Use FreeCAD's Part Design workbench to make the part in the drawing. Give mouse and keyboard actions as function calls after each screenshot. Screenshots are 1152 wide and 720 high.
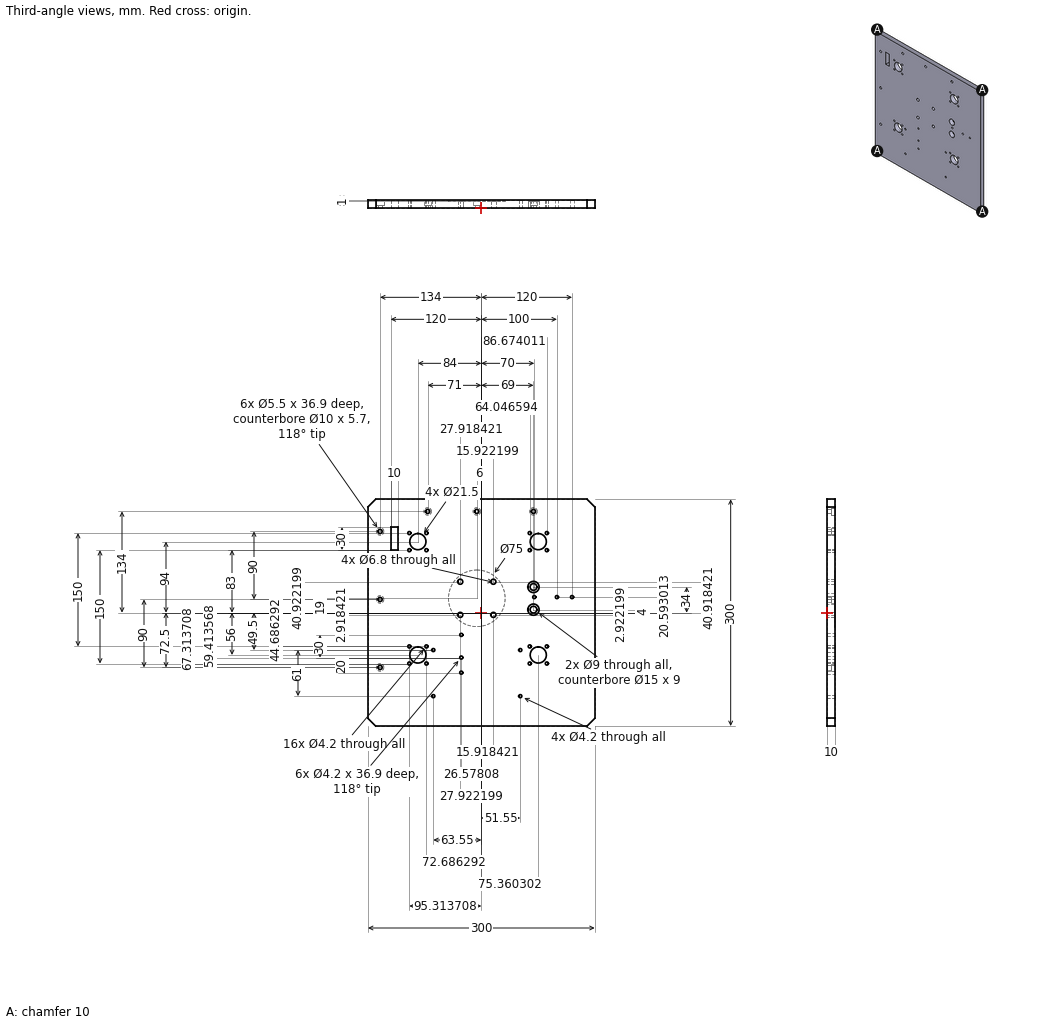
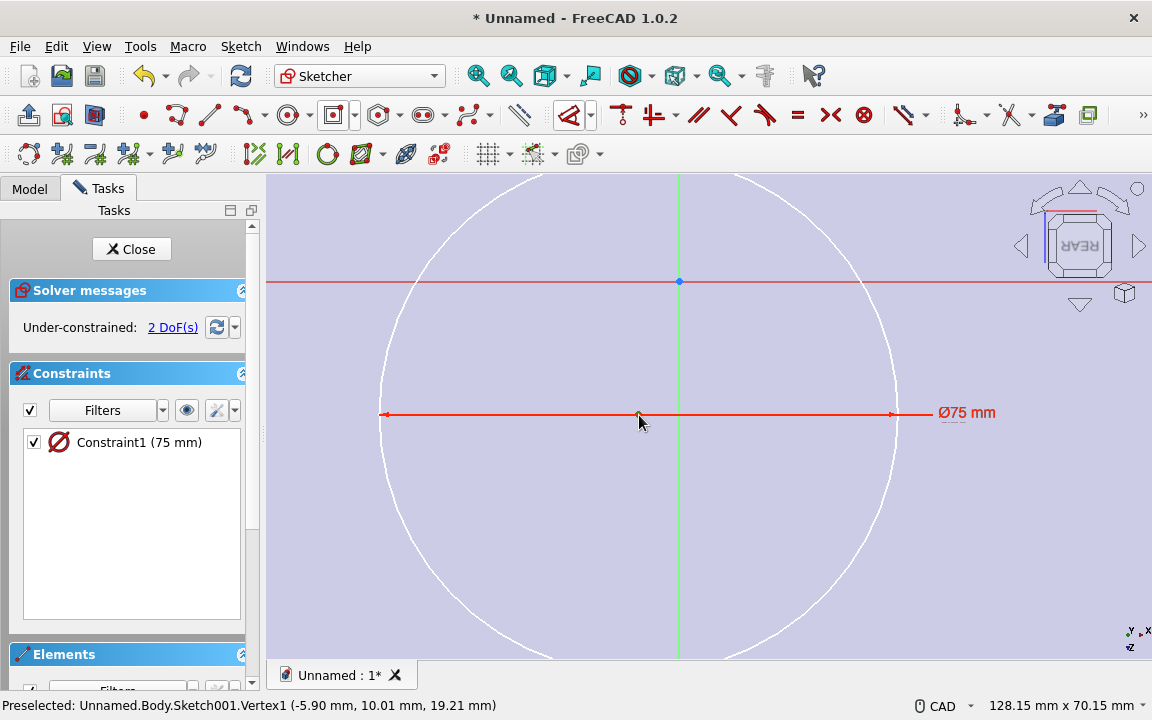
key(l)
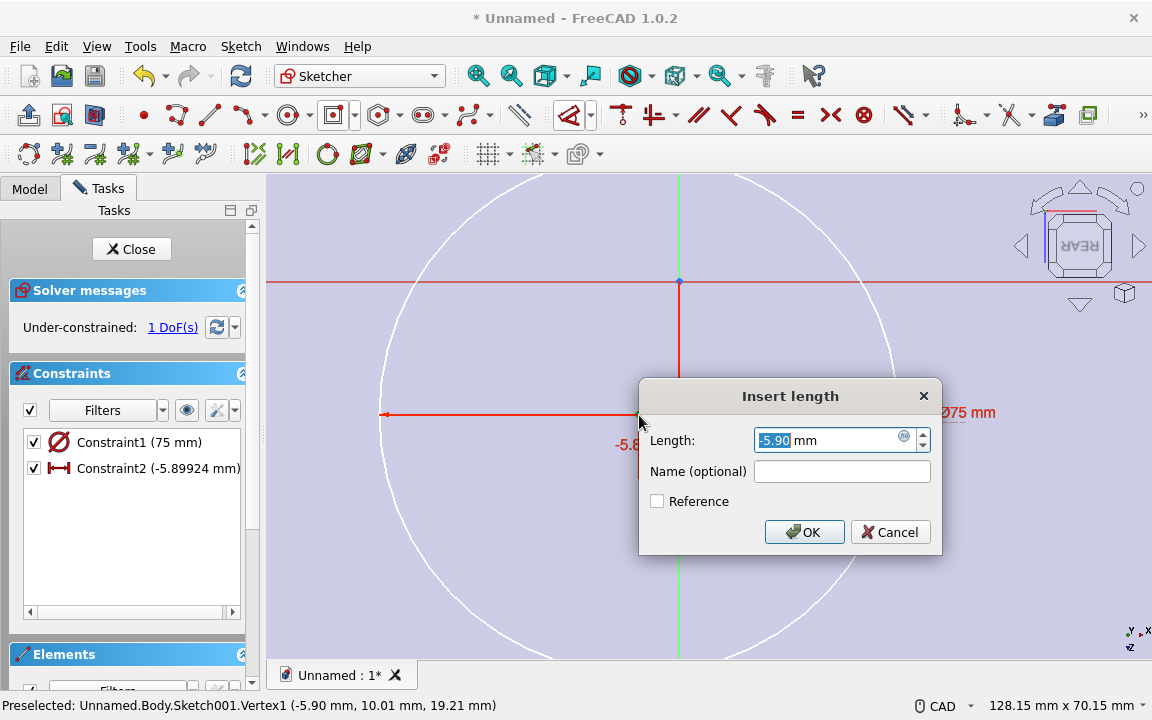
text(-6)
key(Return)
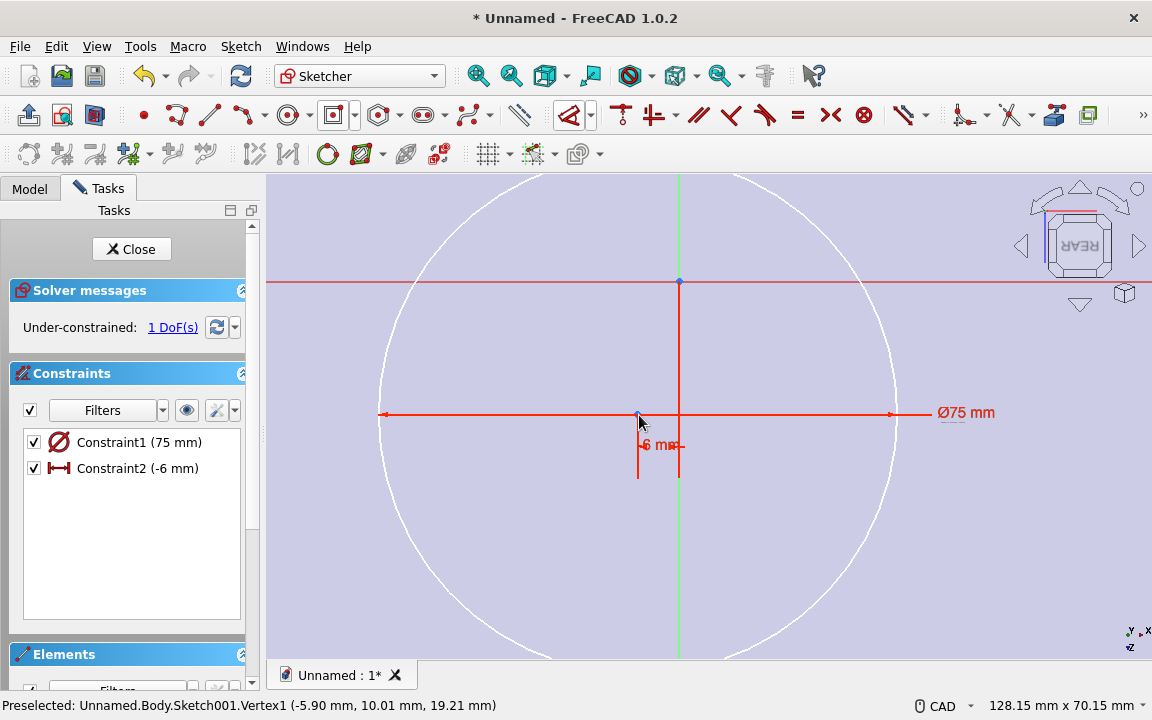
click(638, 415)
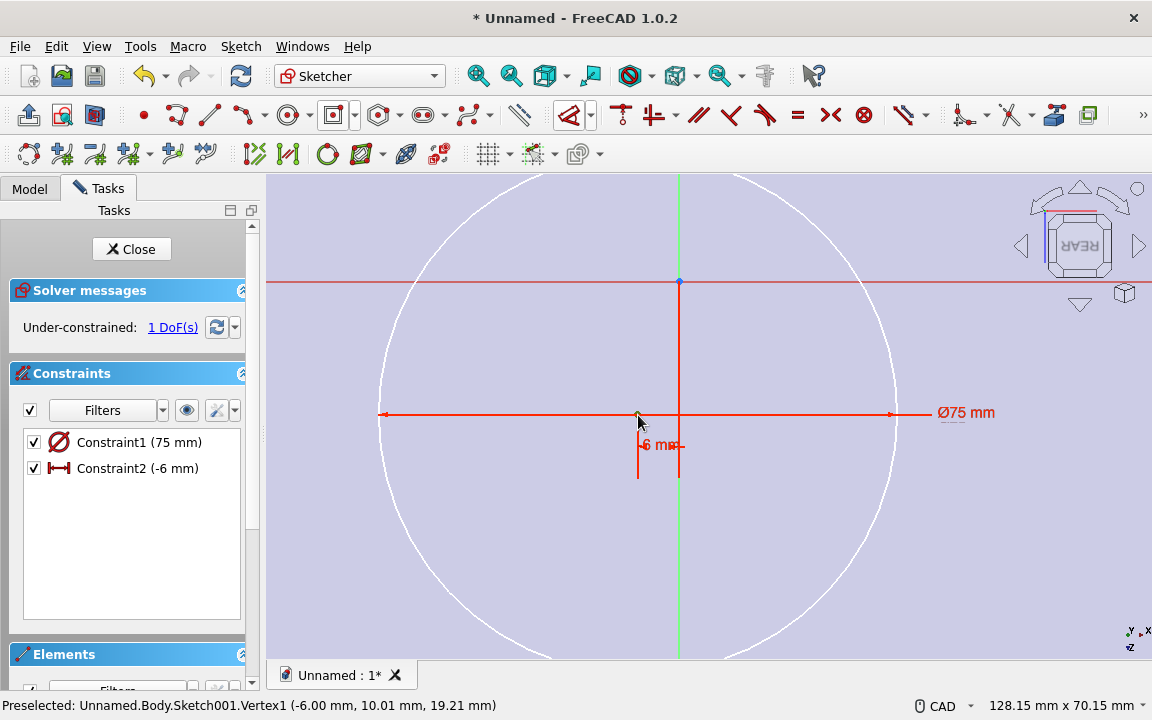
key(i)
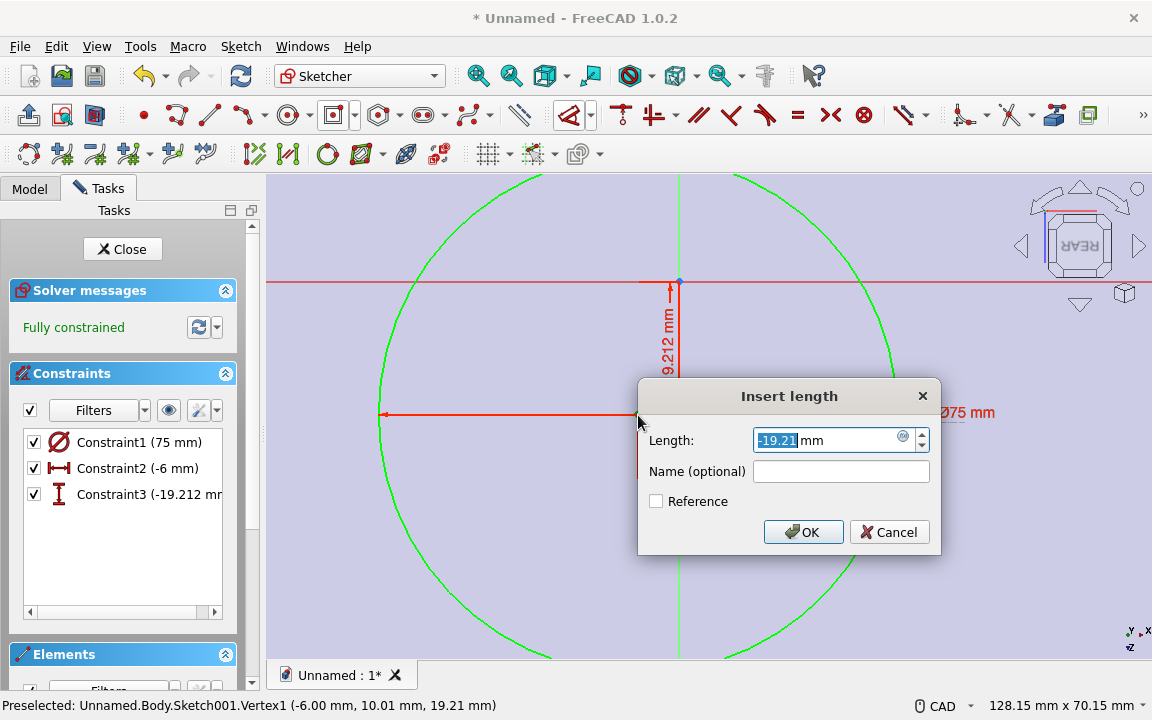
text(-19)
key(Return)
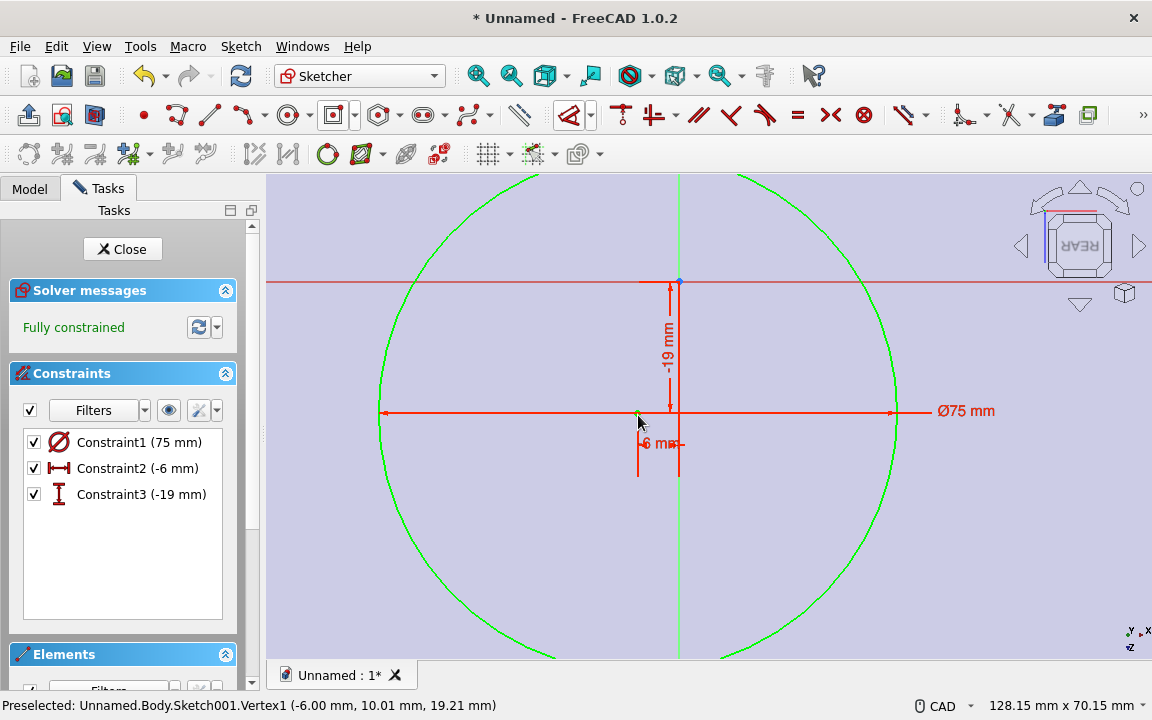
click(123, 249)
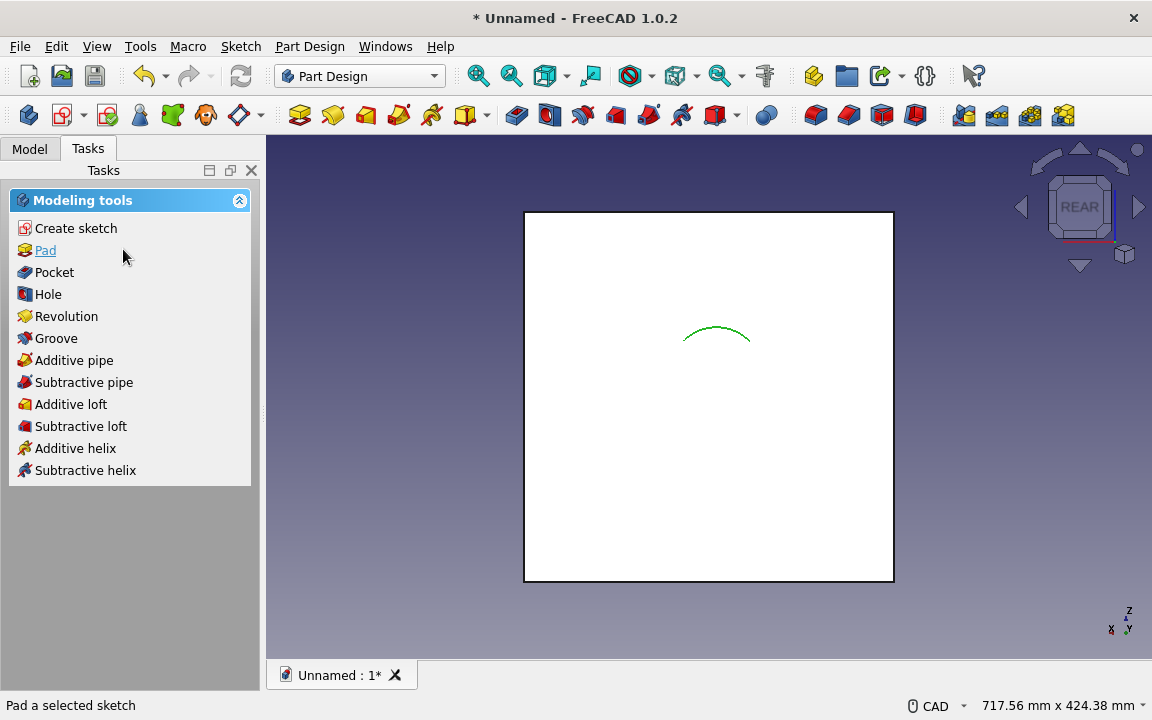
click(517, 116)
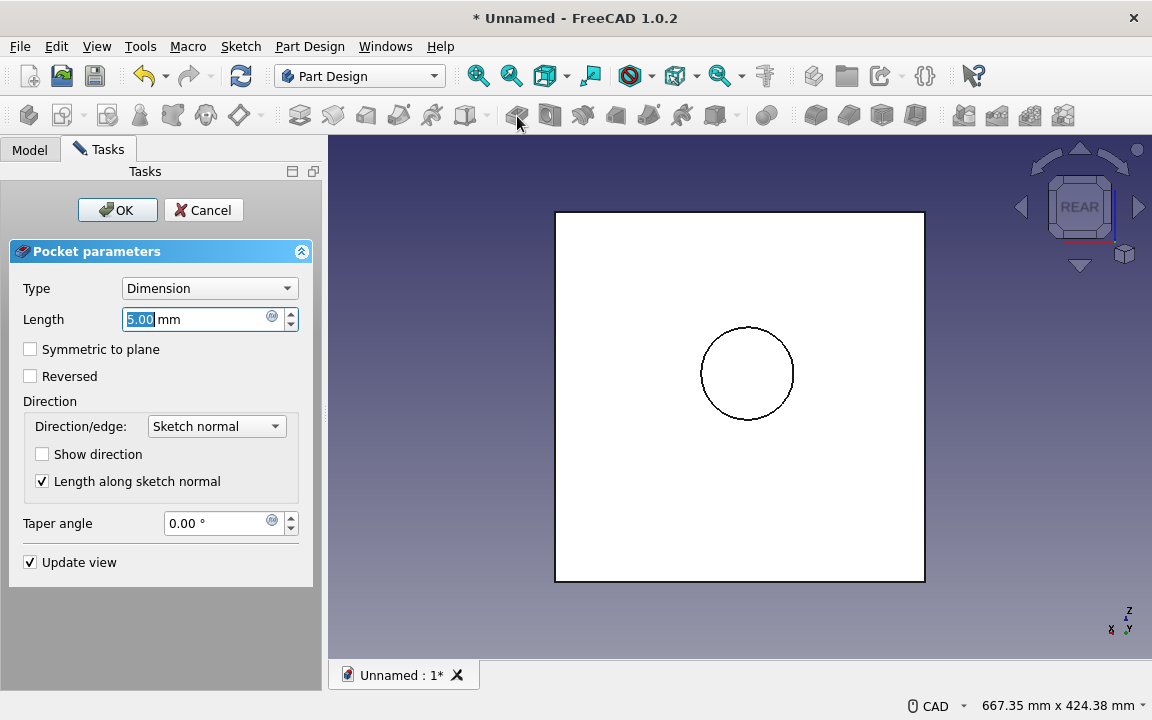
text(1)
key(Tab)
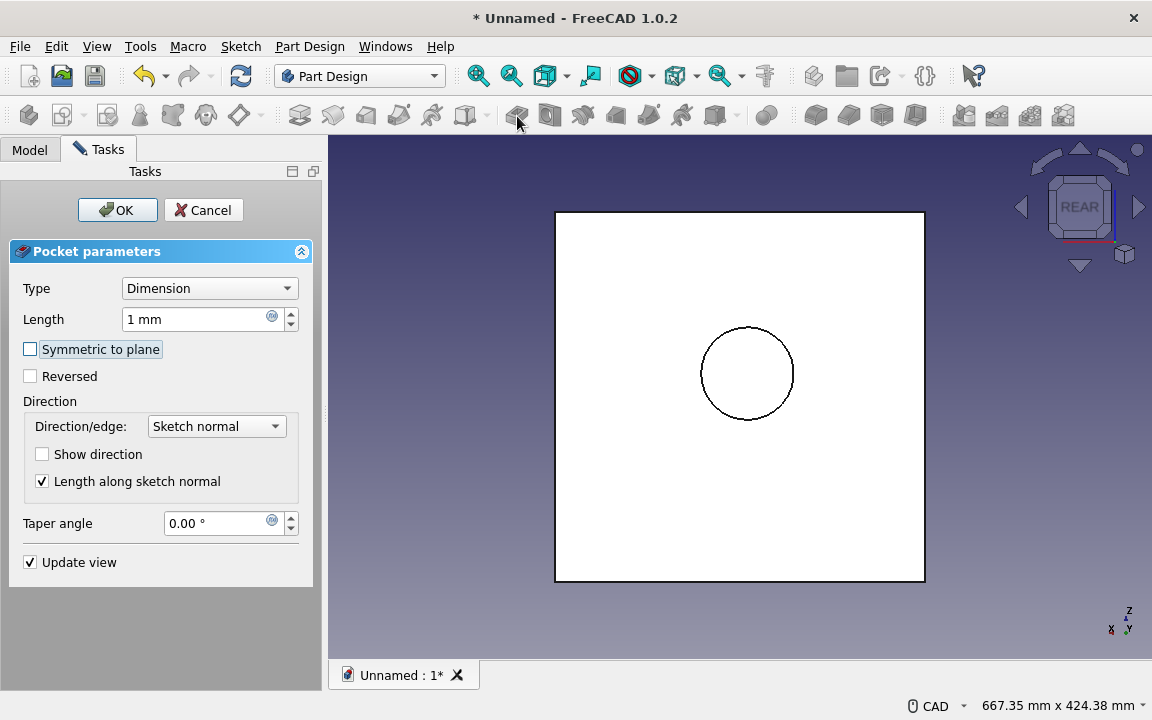
click(118, 210)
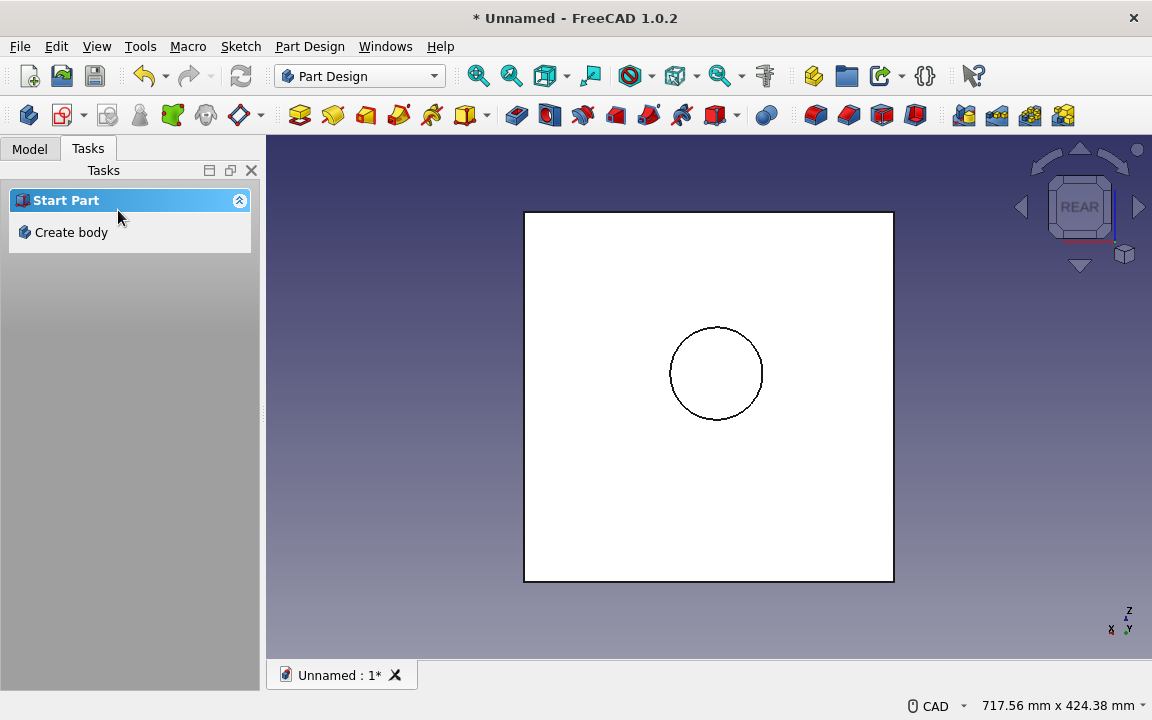
click(656, 502)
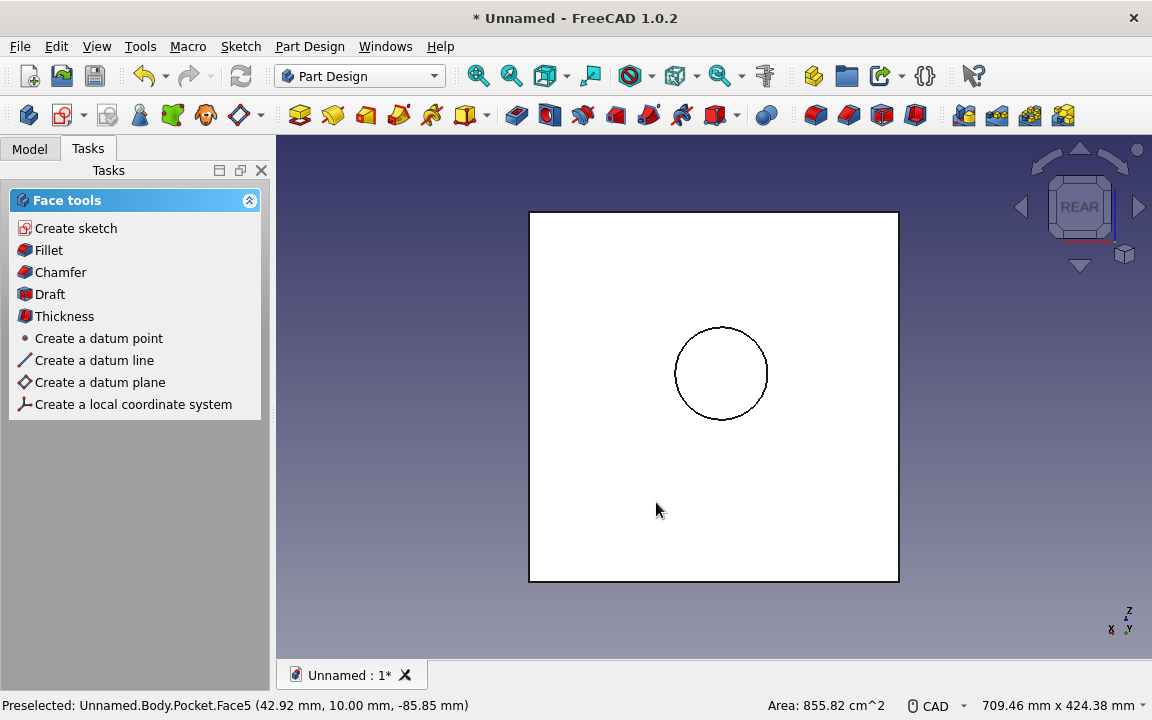
click(62, 116)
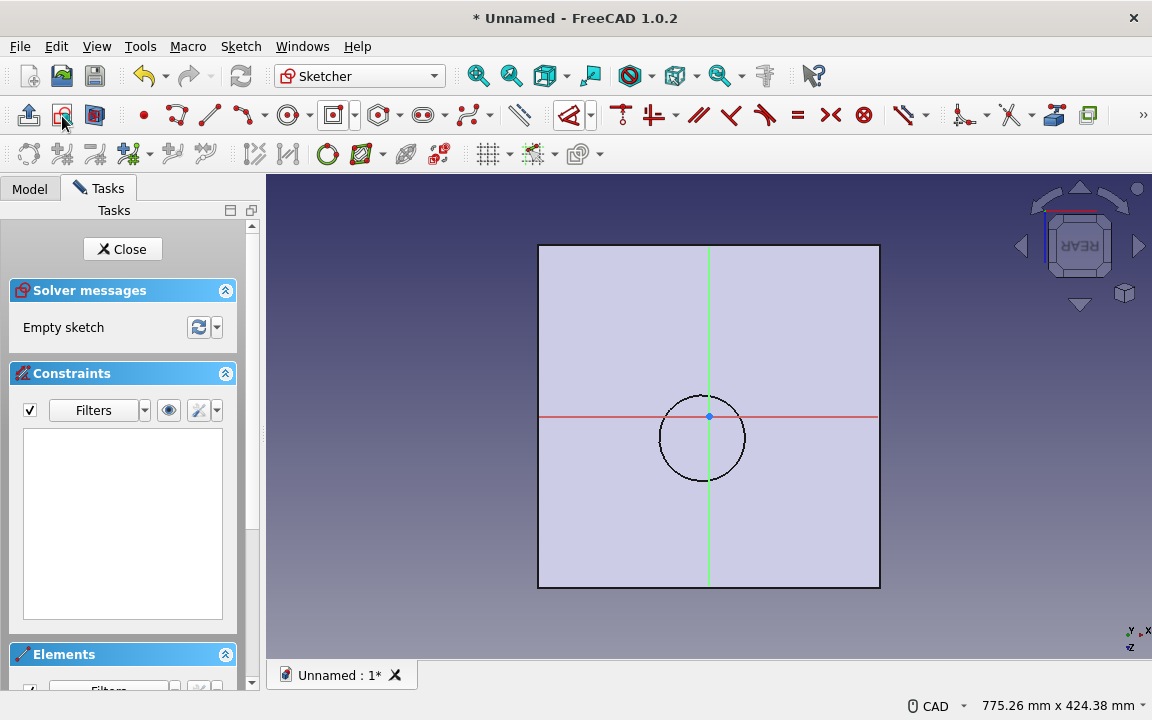
scroll(570, 542, up, 11)